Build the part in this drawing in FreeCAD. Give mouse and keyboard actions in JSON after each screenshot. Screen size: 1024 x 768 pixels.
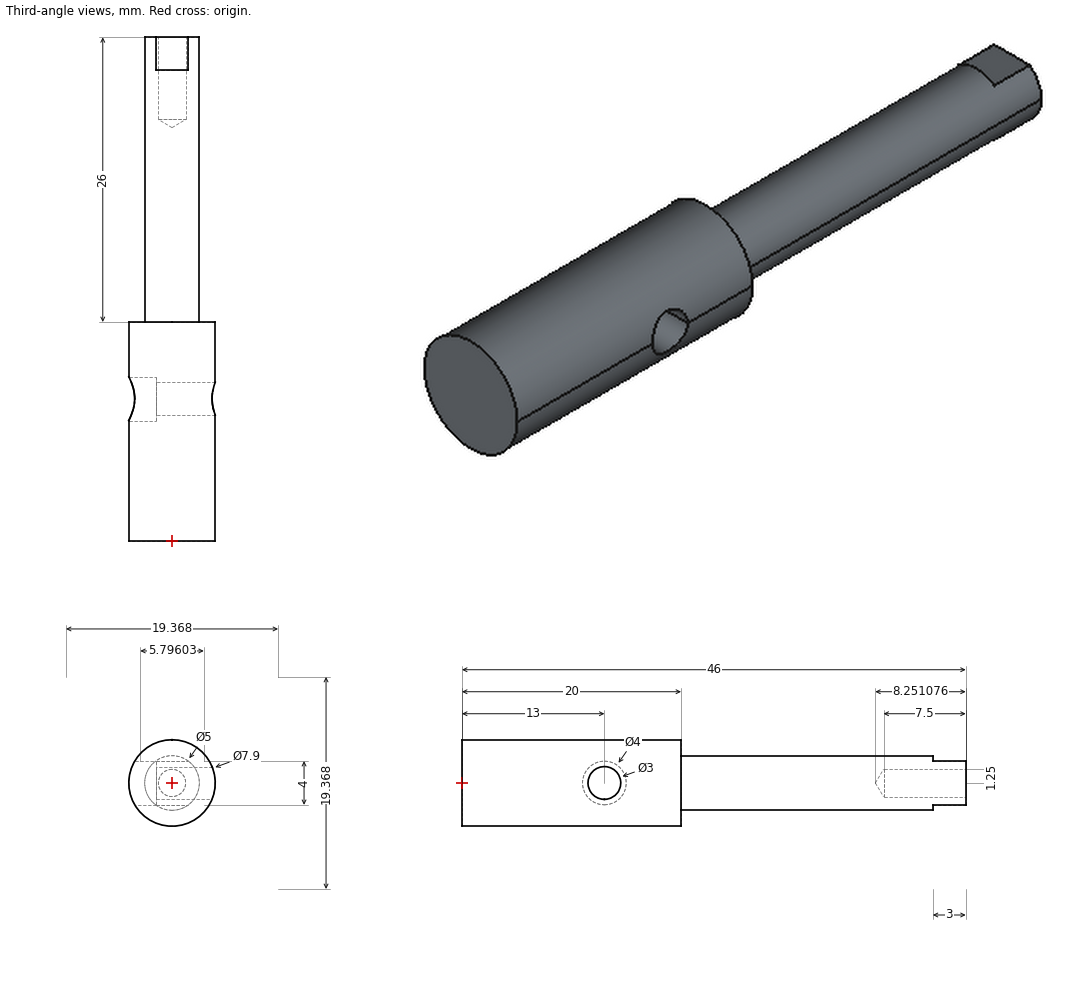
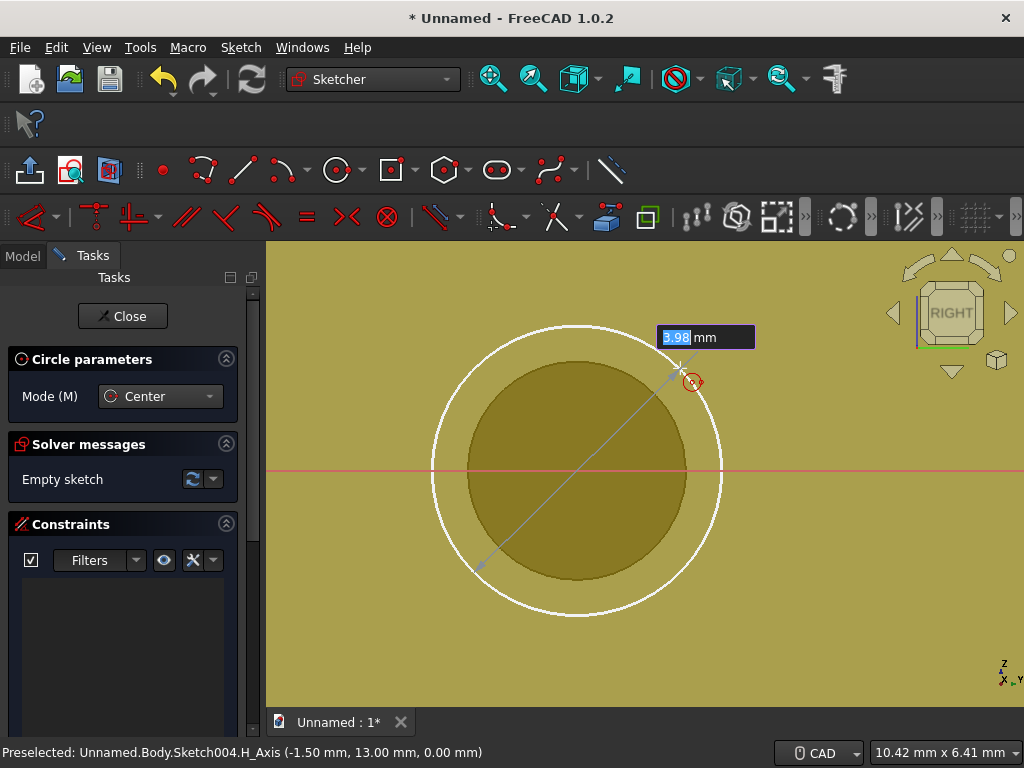
{"action": "type", "text": "4"}
{"action": "key", "text": "Return"}
{"action": "key", "text": "Escape"}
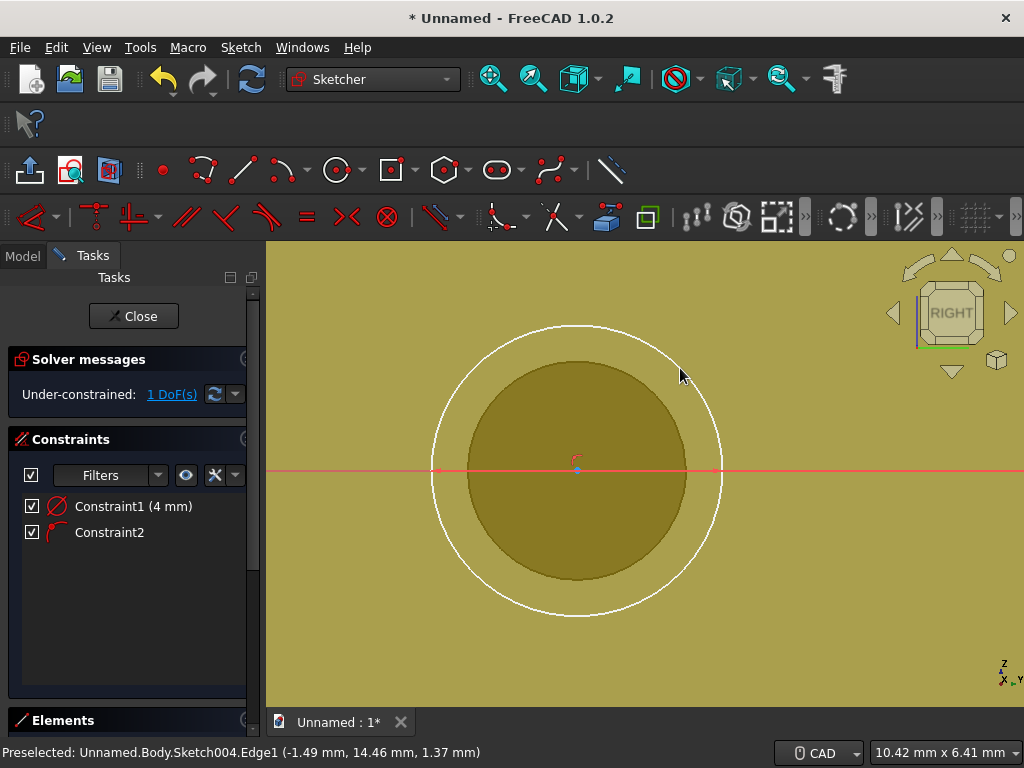
{"action": "left_click", "coordinate": [32, 218]}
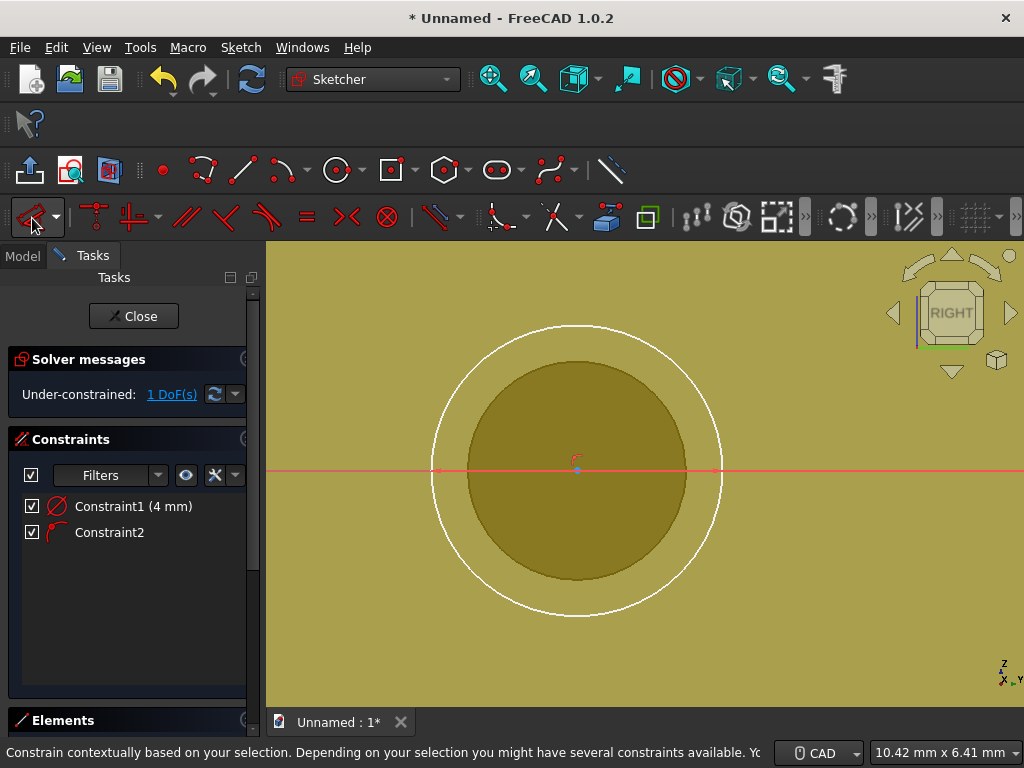
{"action": "left_click", "coordinate": [577, 471]}
{"action": "left_click", "coordinate": [370, 505]}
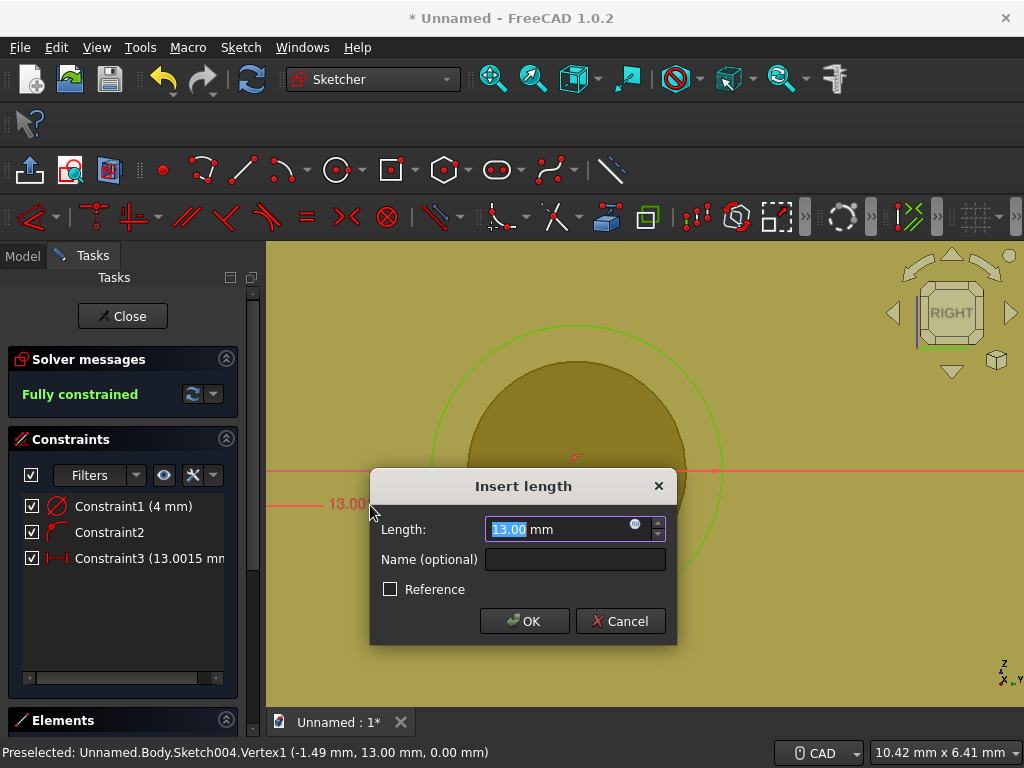
{"action": "type", "text": "13"}
{"action": "key", "text": "Return"}
{"action": "key", "text": "Escape"}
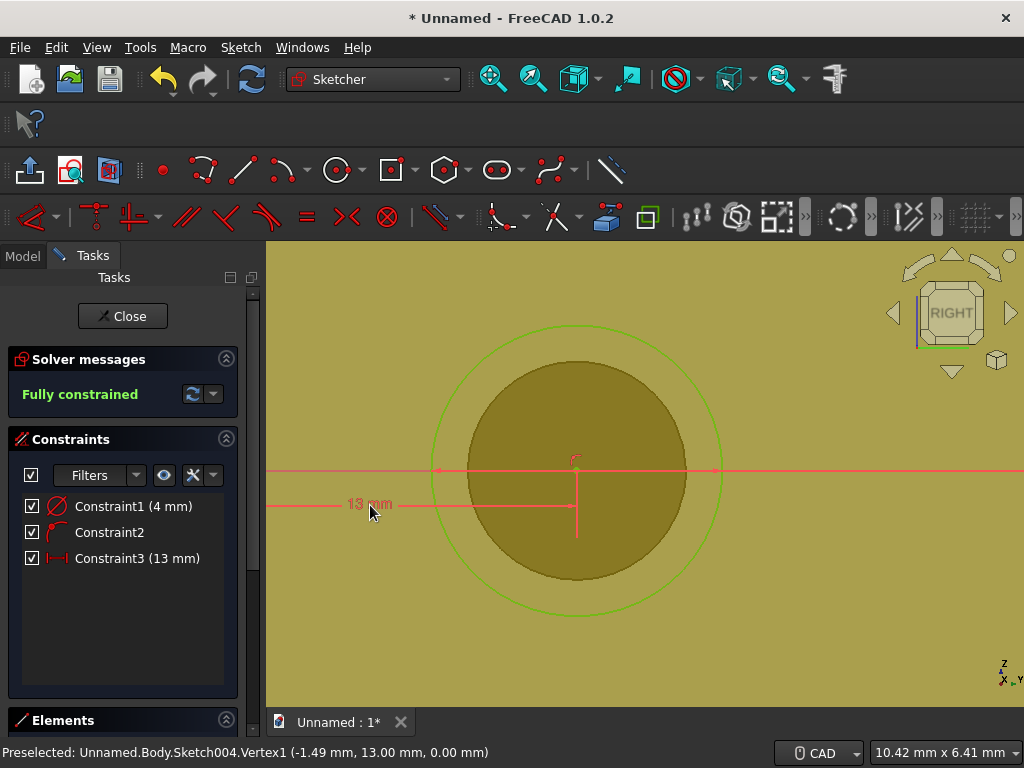
{"action": "left_click", "coordinate": [123, 316]}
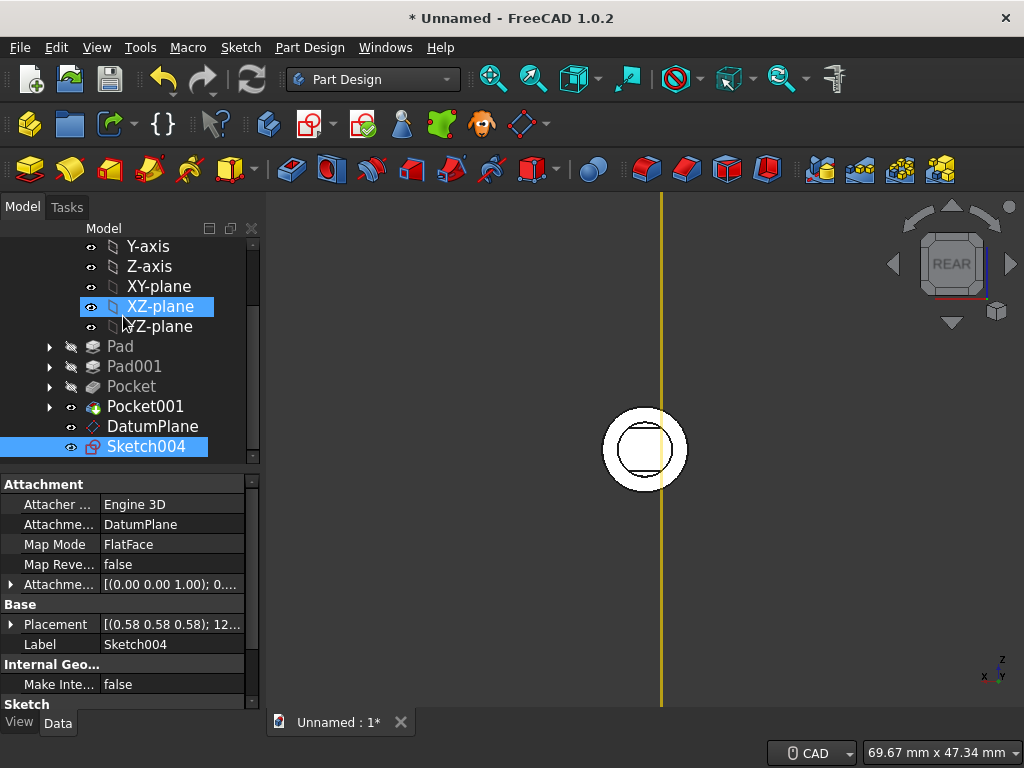
{"action": "left_click", "coordinate": [292, 170]}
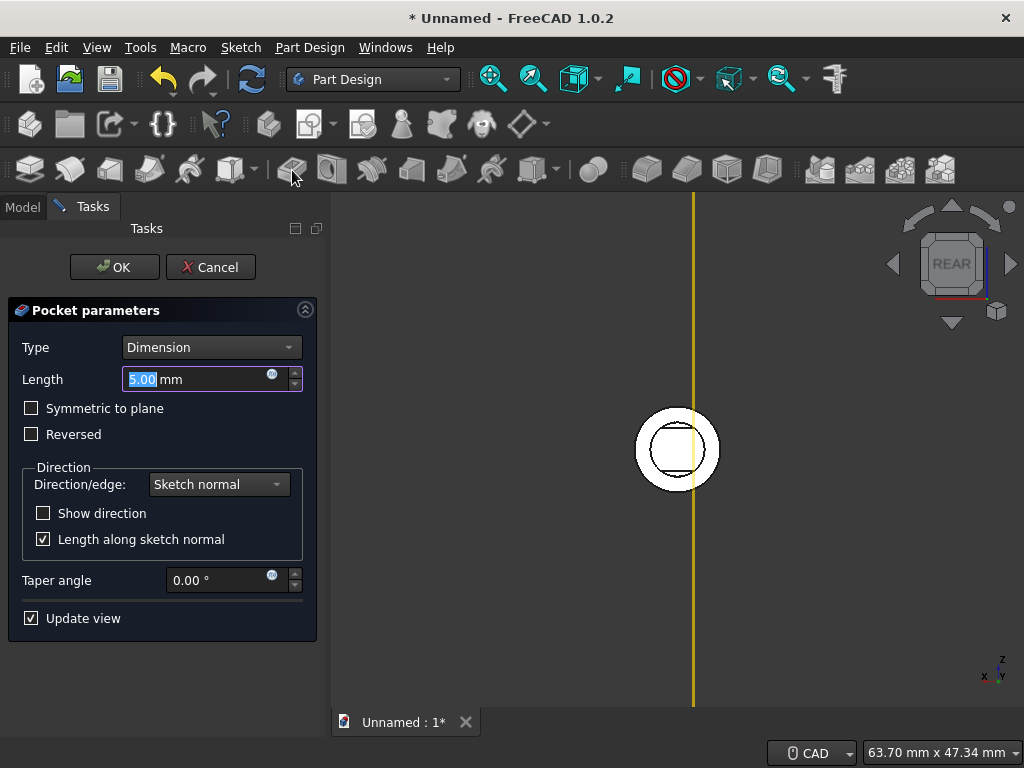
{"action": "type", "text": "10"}
{"action": "key", "text": "Tab"}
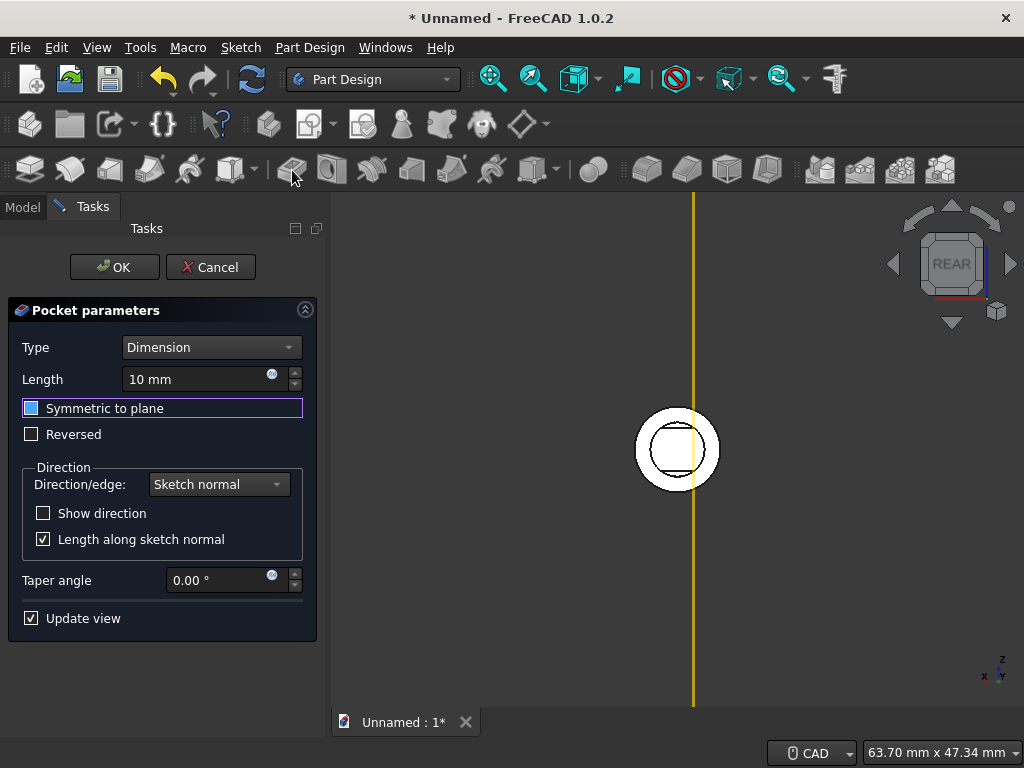
{"action": "left_click", "coordinate": [115, 267]}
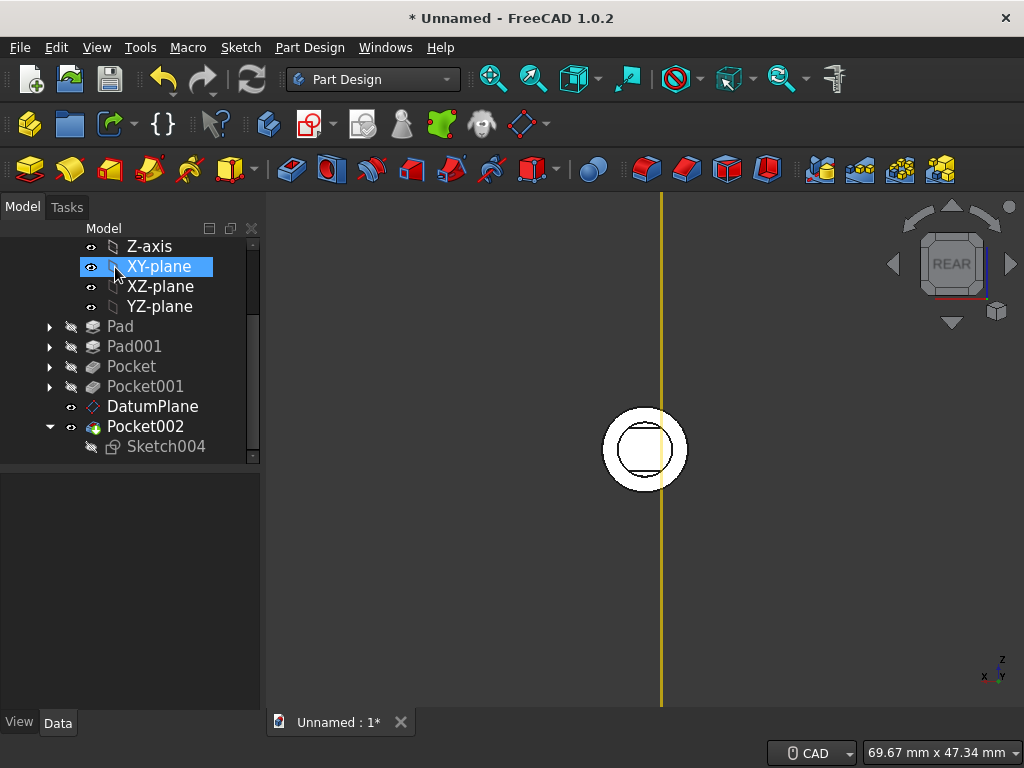
{"action": "left_click", "coordinate": [116, 407]}
{"action": "key", "text": "space"}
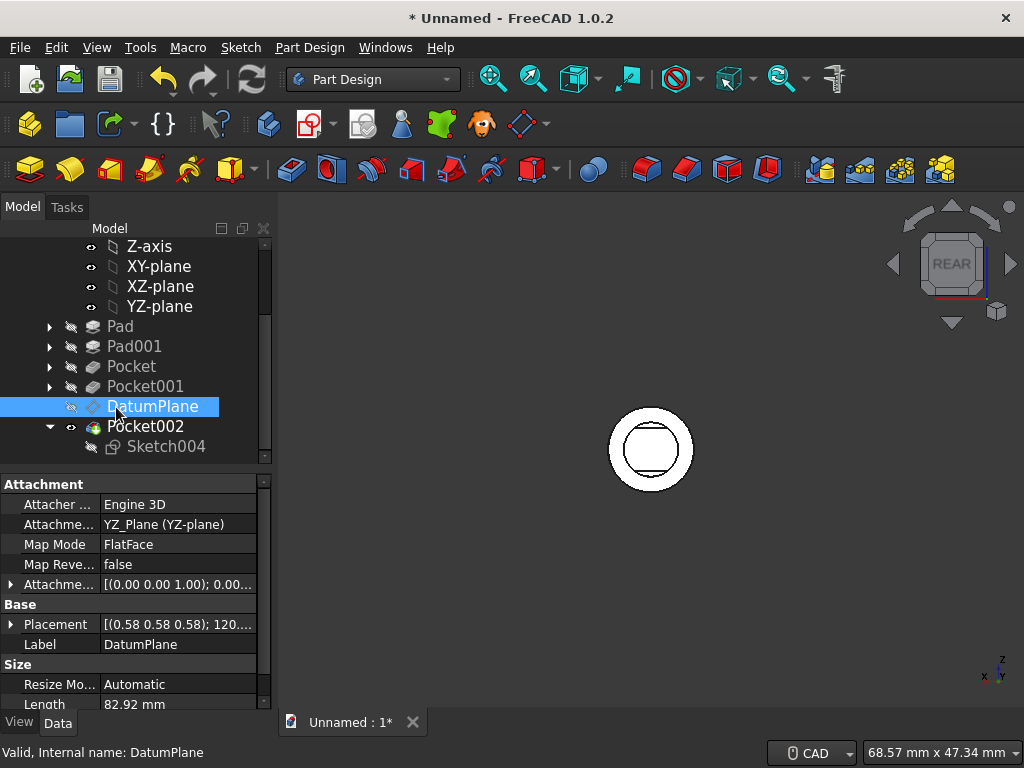
{"action": "left_click", "coordinate": [494, 80]}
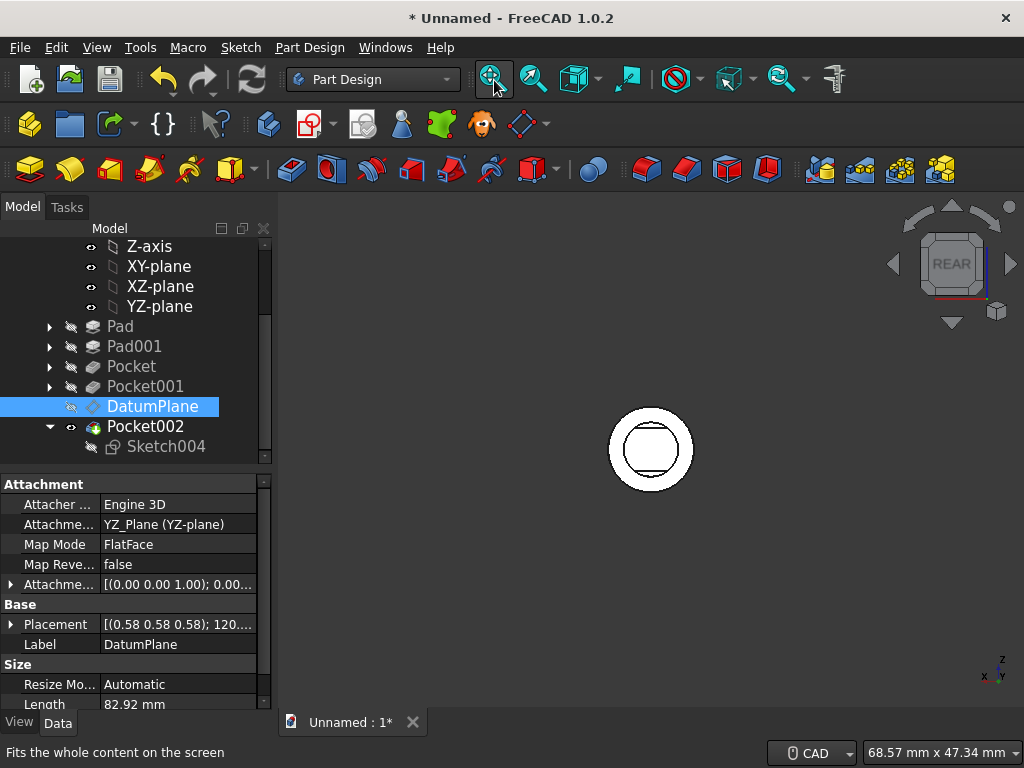
{"action": "left_click", "coordinate": [318, 667]}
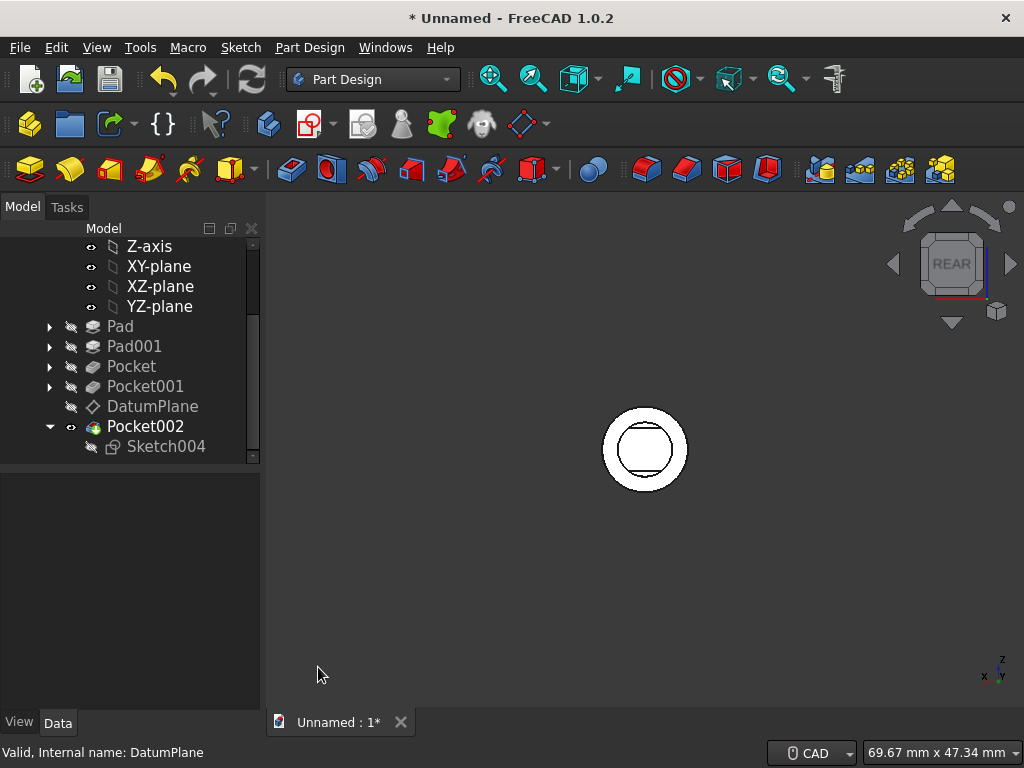
{"action": "left_click", "coordinate": [310, 124]}